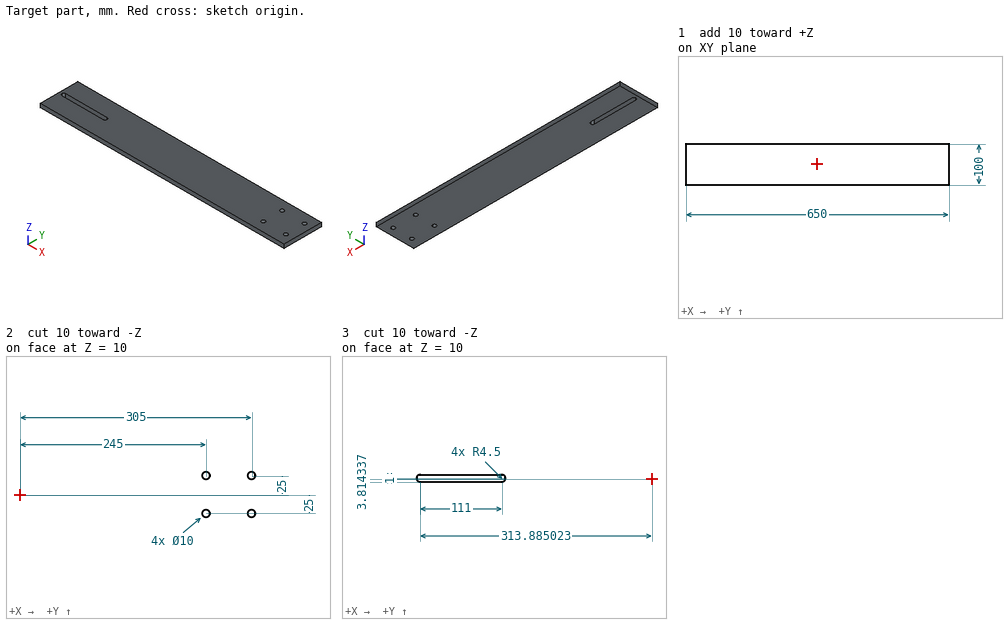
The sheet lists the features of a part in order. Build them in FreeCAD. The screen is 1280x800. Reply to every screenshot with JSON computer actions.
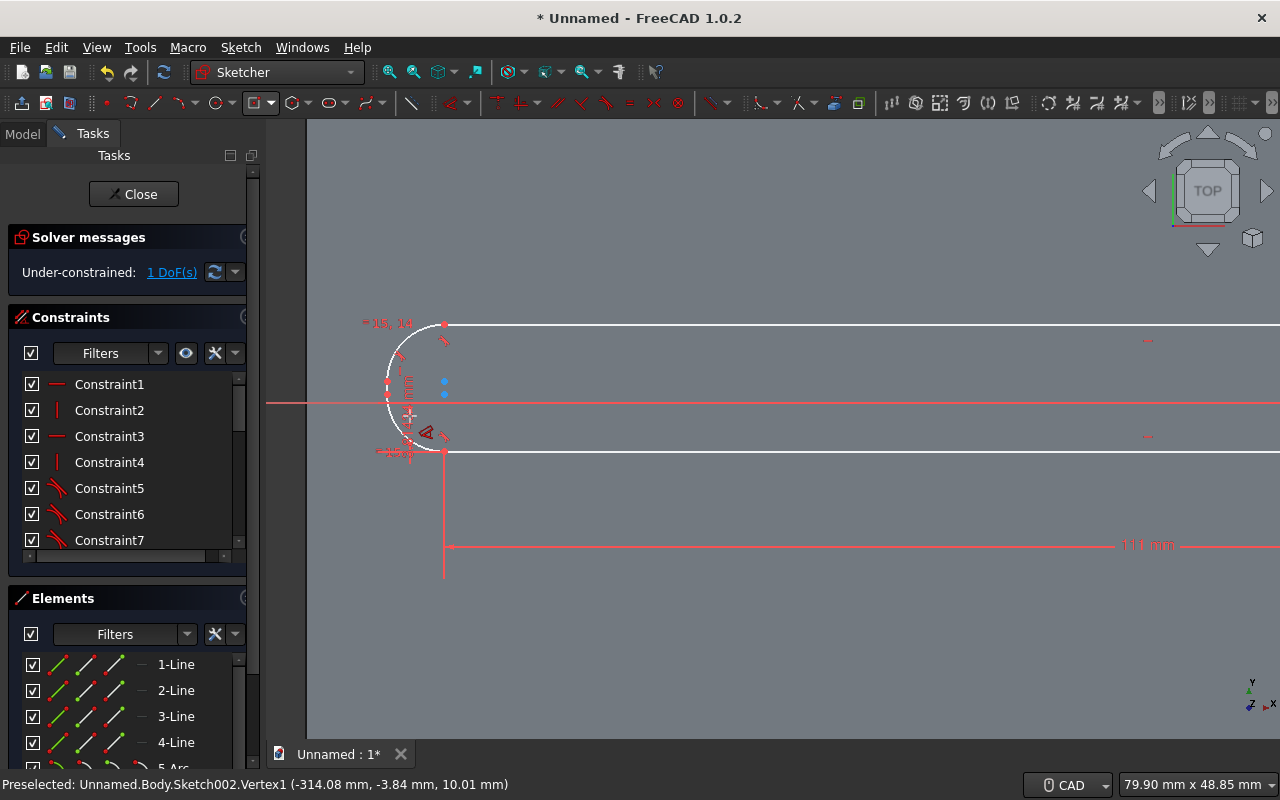
{"action": "left_click", "coordinate": [444, 452]}
{"action": "left_click", "coordinate": [780, 486]}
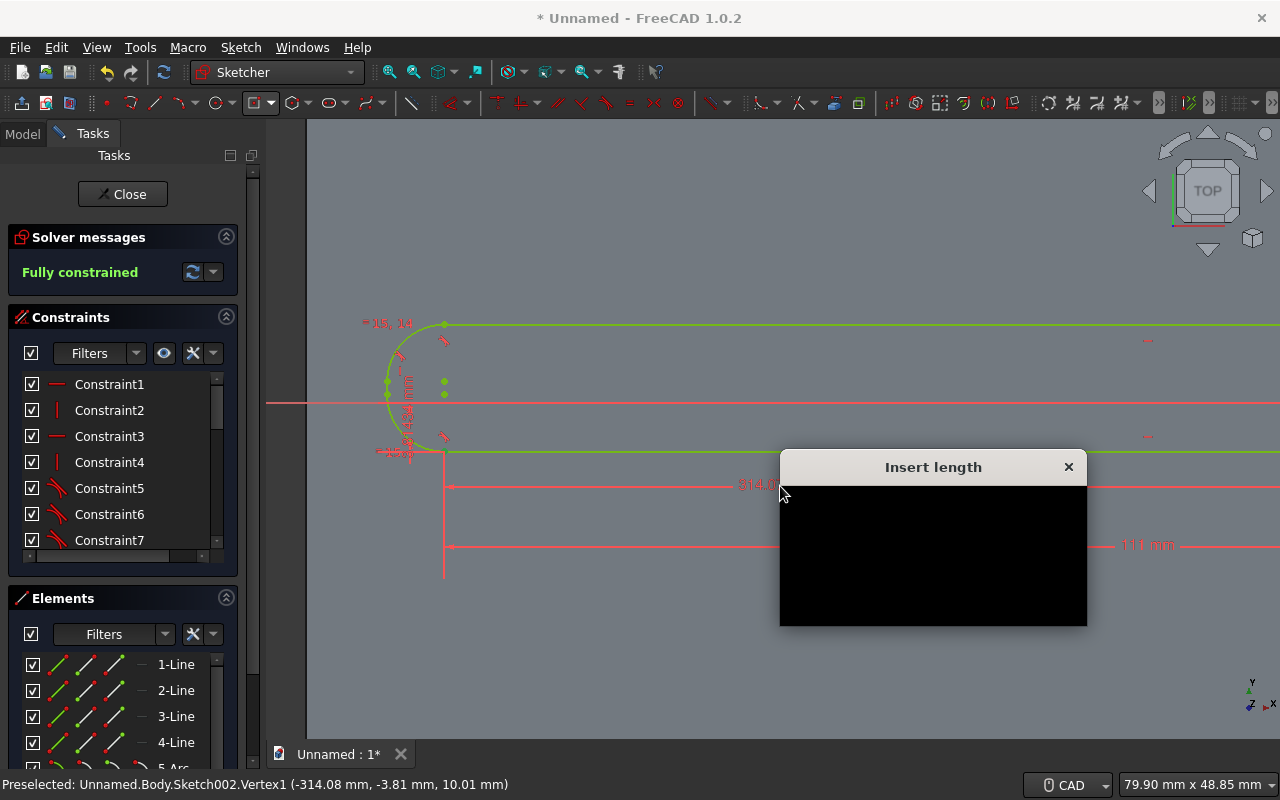
{"action": "type", "text": "313.885023"}
{"action": "key", "text": "Return"}
{"action": "key", "text": "Escape"}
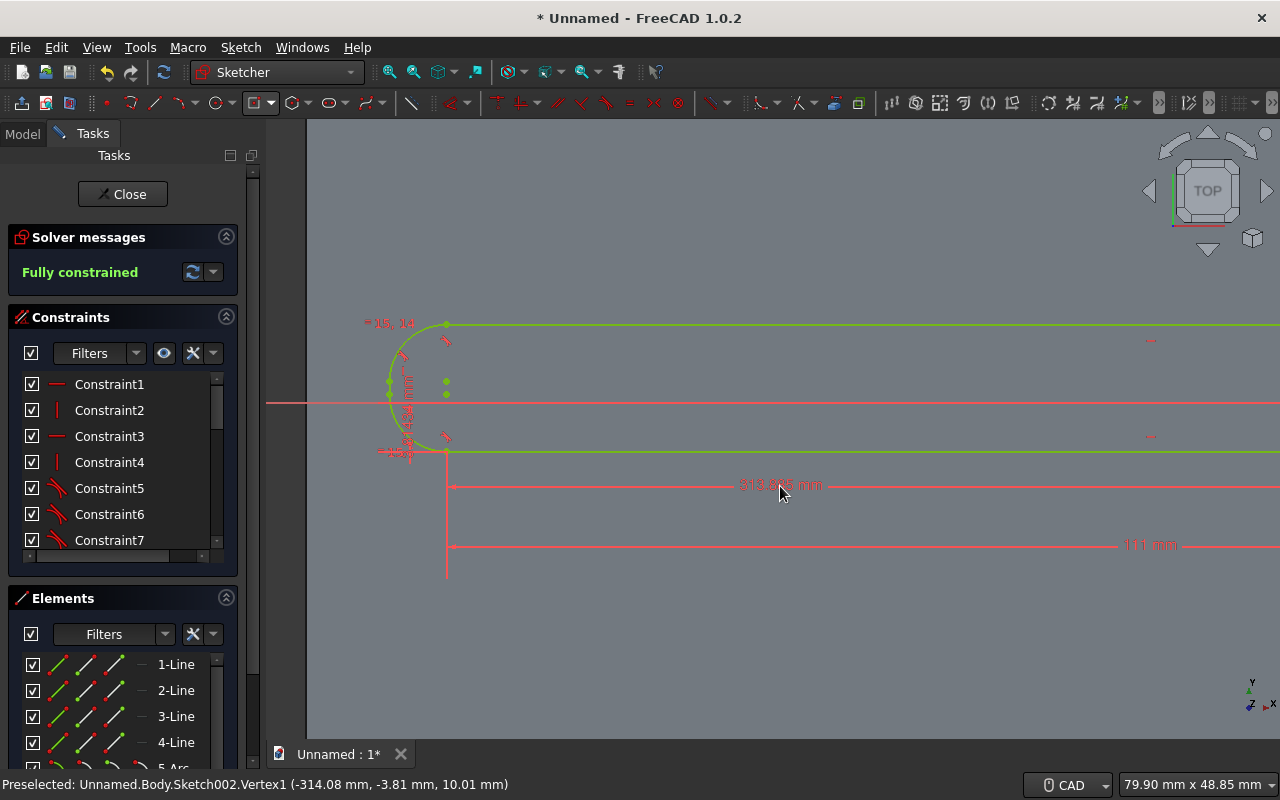
{"action": "left_click", "coordinate": [123, 194]}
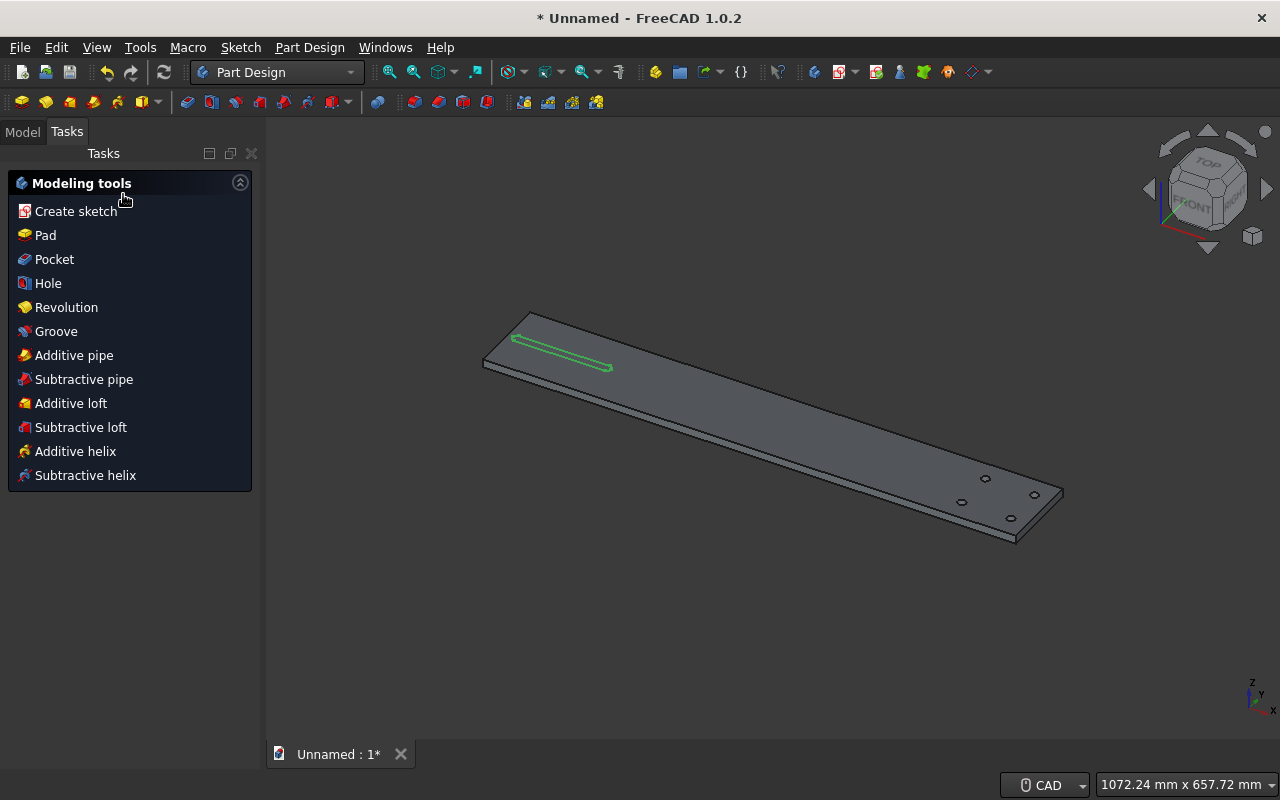
{"action": "left_click", "coordinate": [188, 102]}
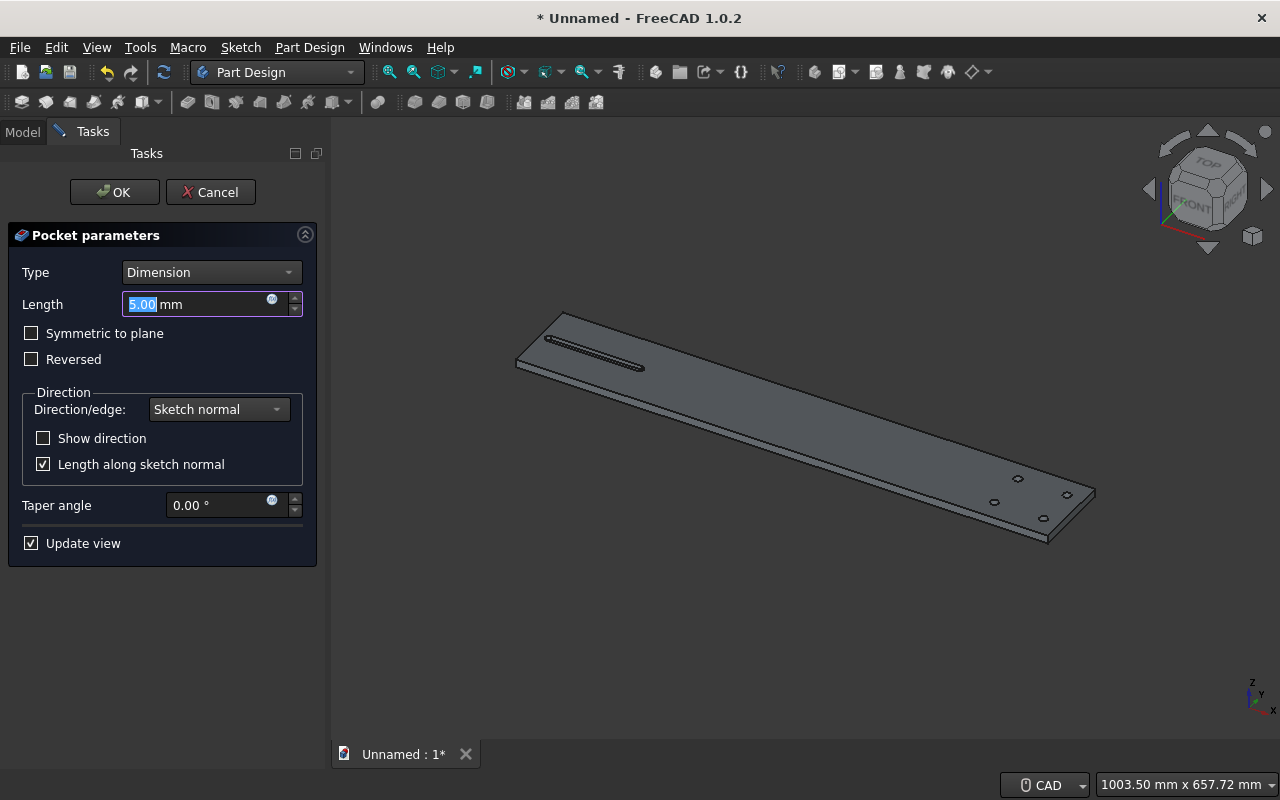
{"action": "type", "text": "10"}
{"action": "key", "text": "Tab"}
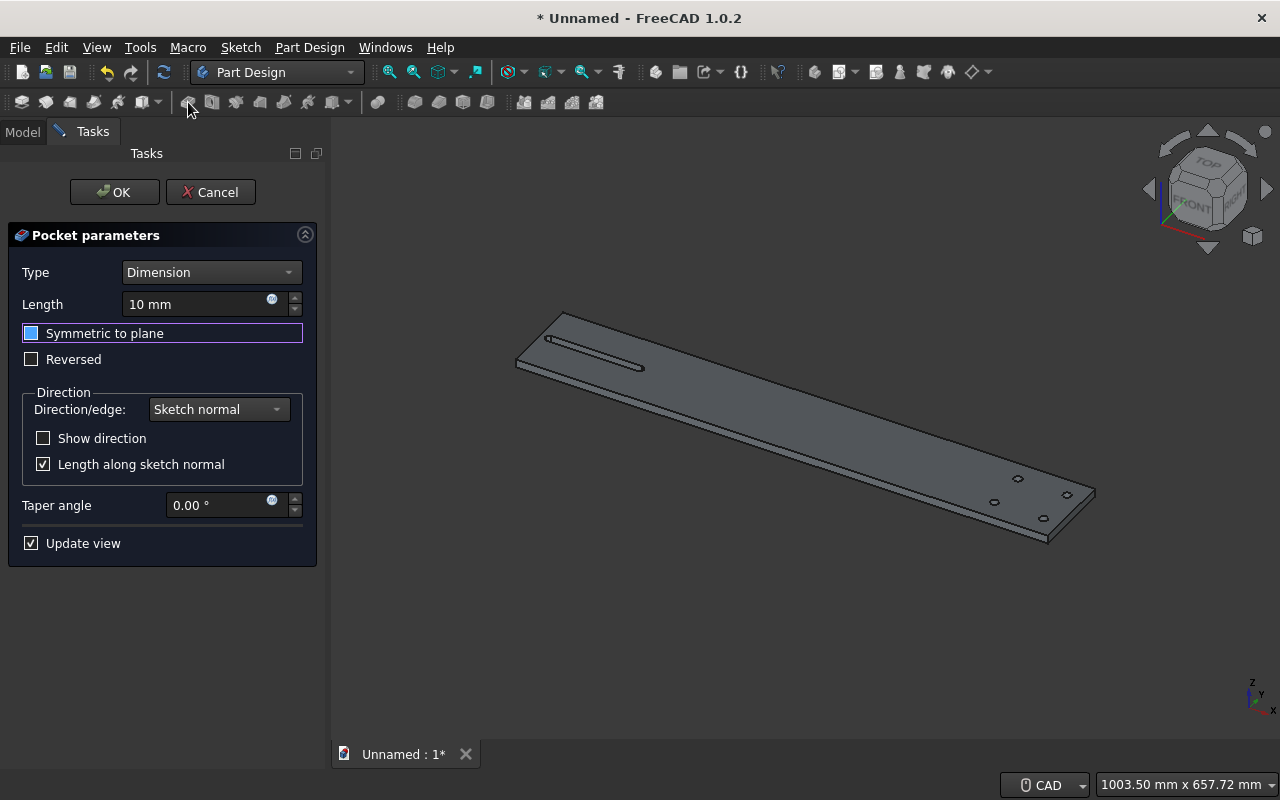
{"action": "left_click", "coordinate": [115, 192]}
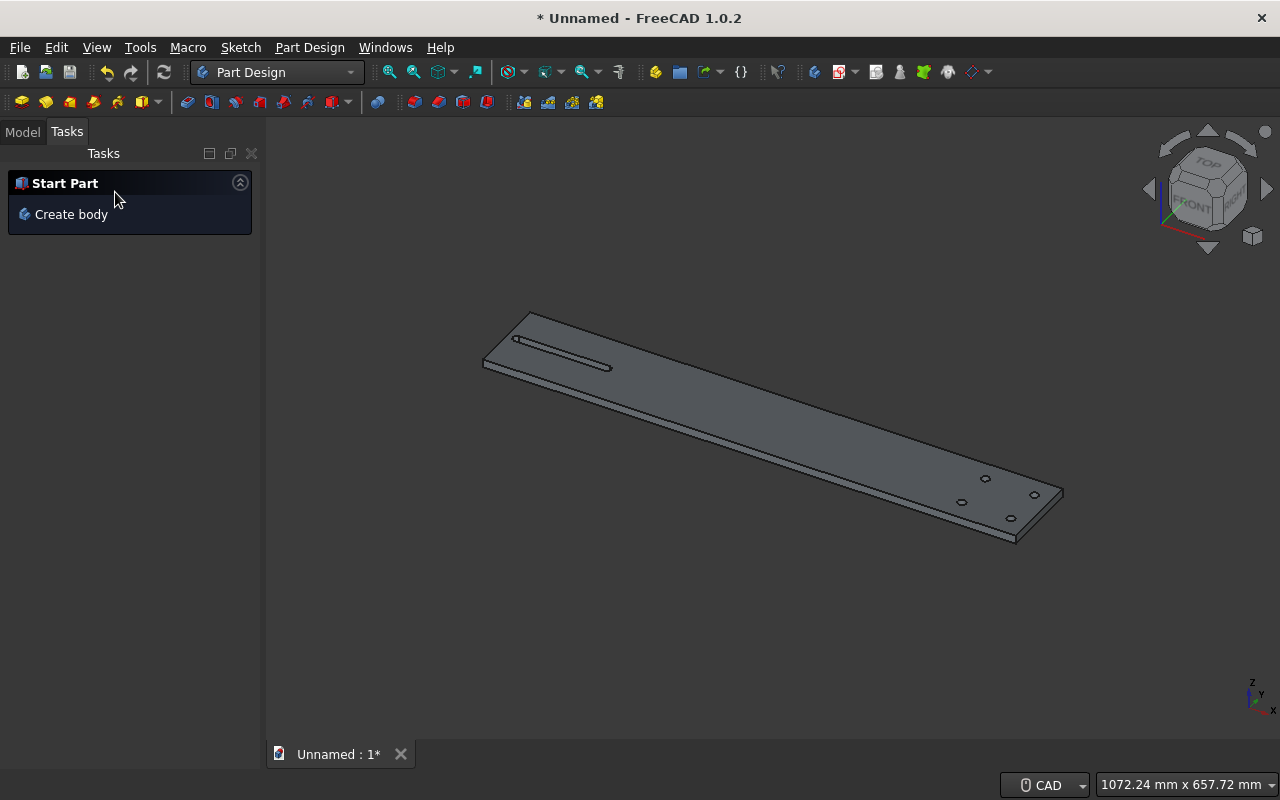
{"action": "key", "text": "0"}